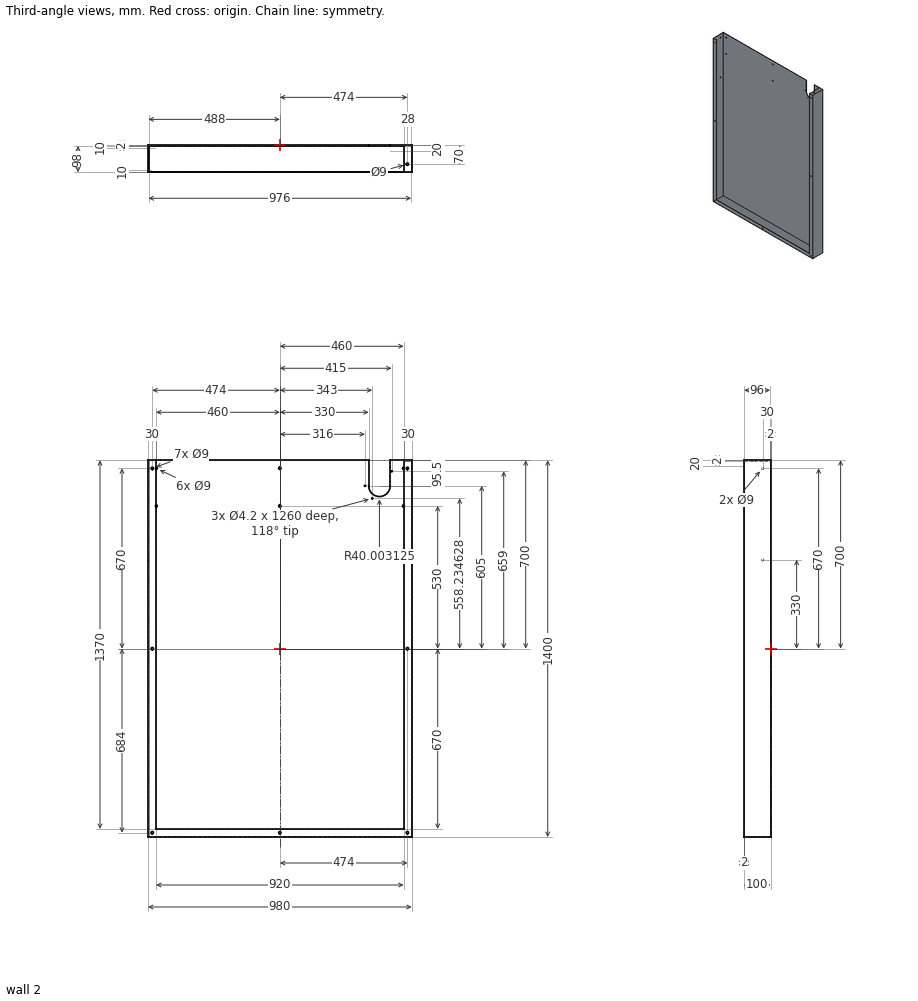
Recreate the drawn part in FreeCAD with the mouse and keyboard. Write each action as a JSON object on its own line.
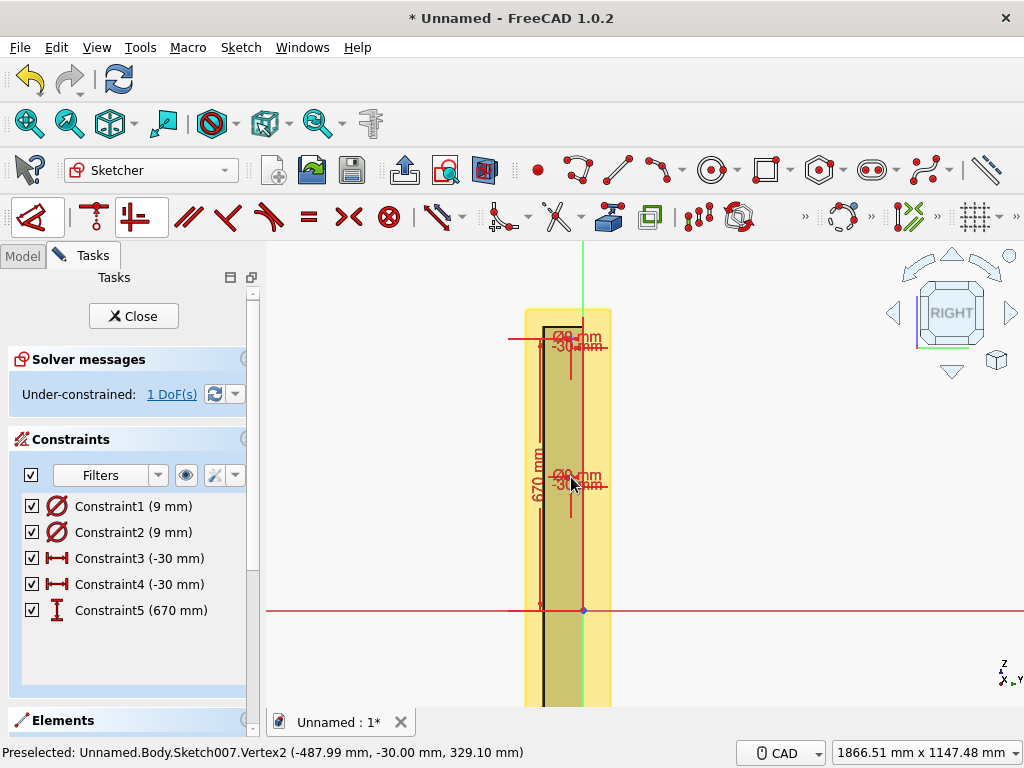
{"action": "key", "text": "i"}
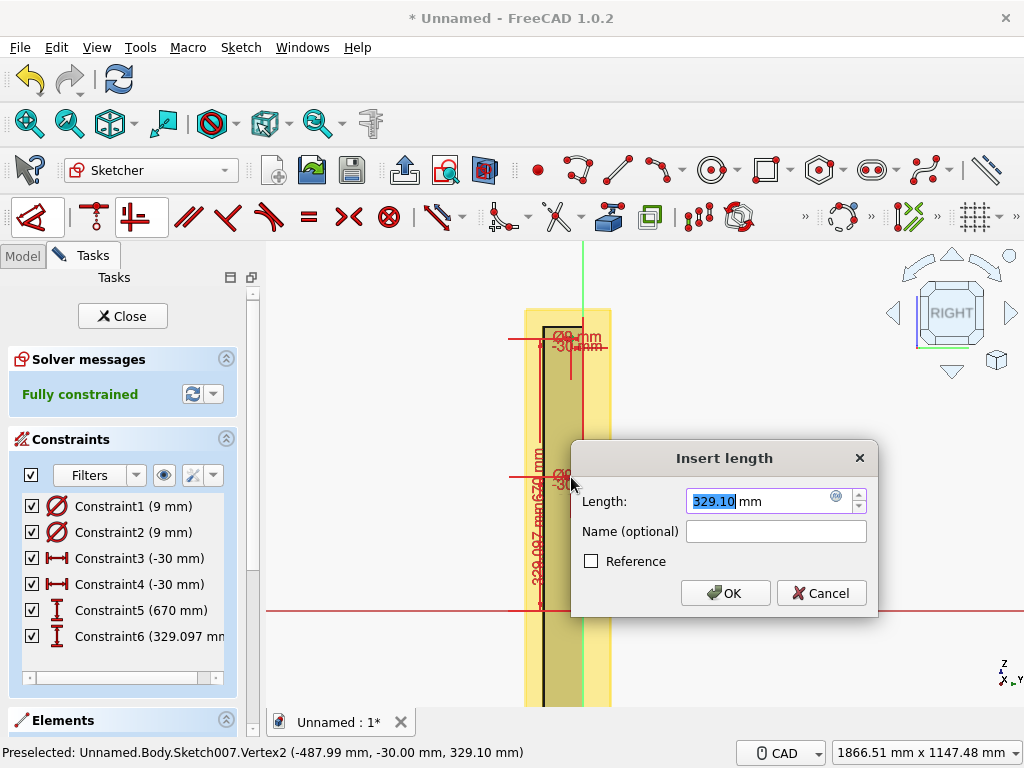
{"action": "type", "text": "330"}
{"action": "key", "text": "Return"}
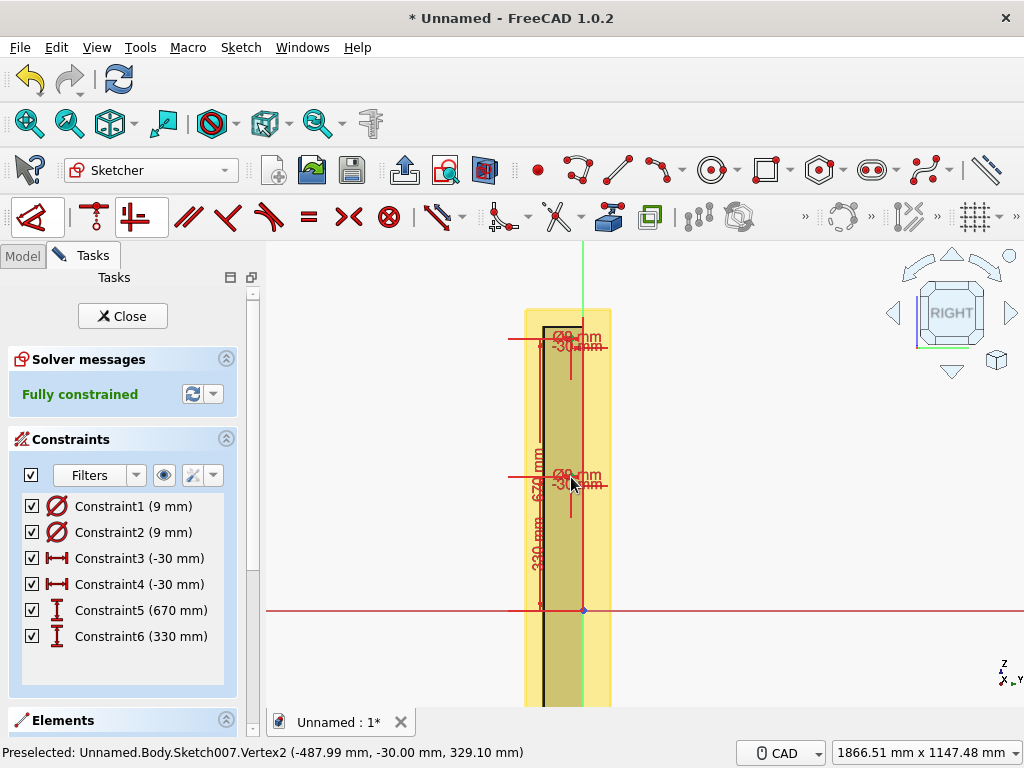
{"action": "left_click", "coordinate": [123, 316]}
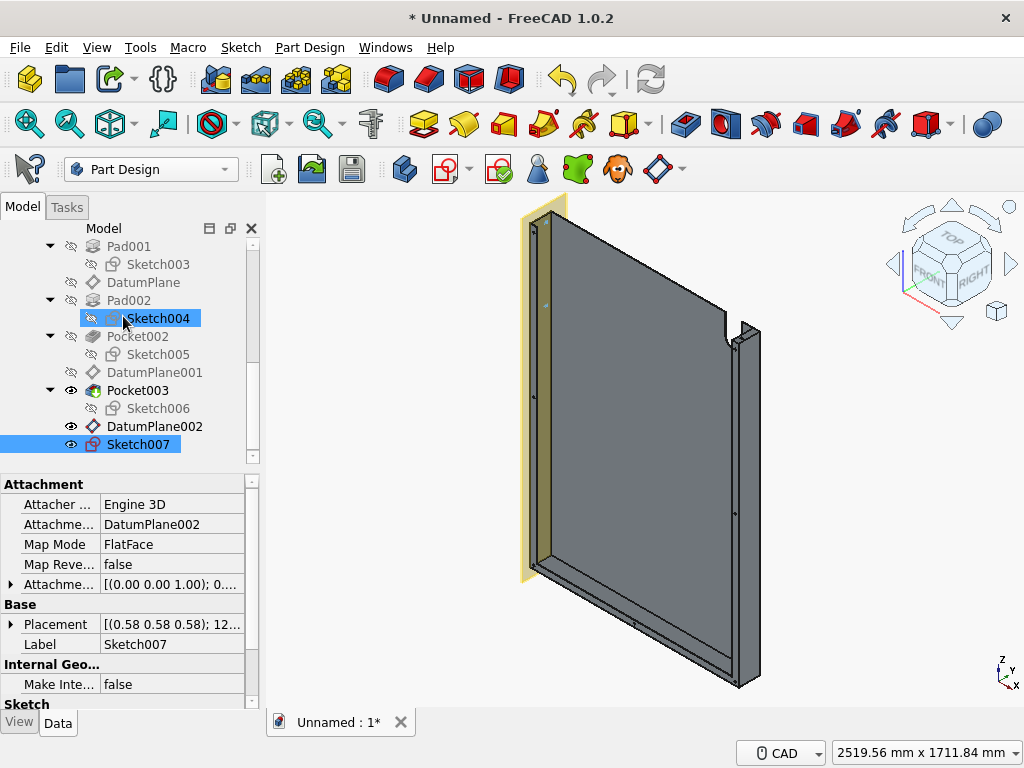
{"action": "left_click", "coordinate": [686, 124]}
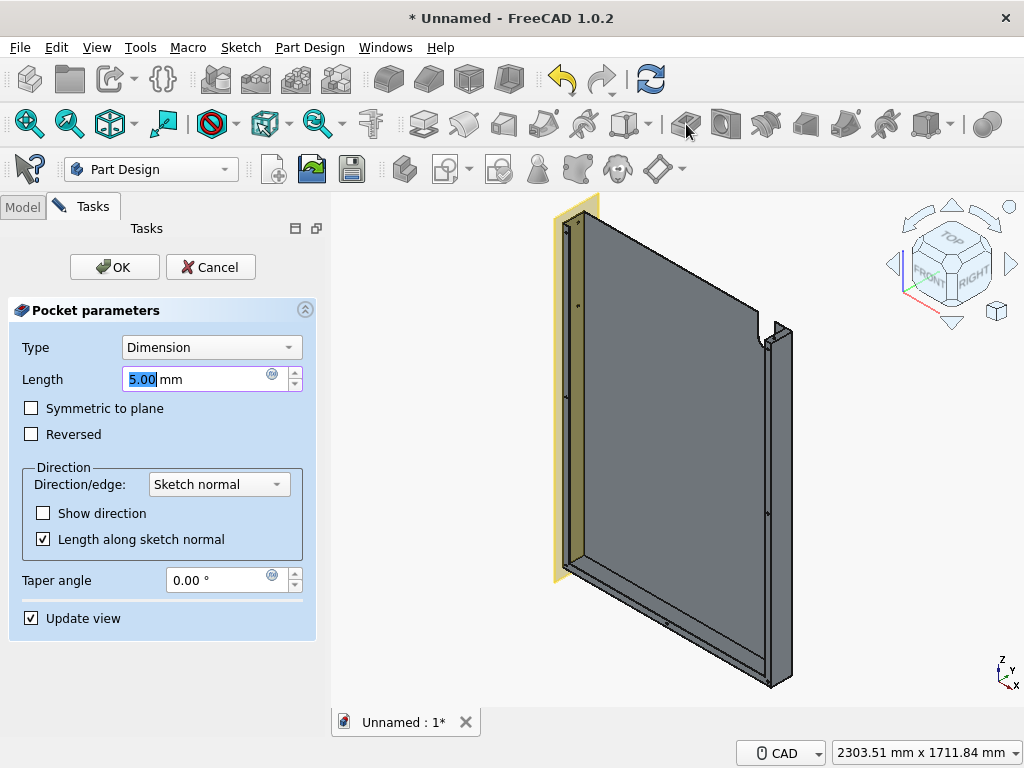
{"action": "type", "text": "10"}
{"action": "key", "text": "Tab"}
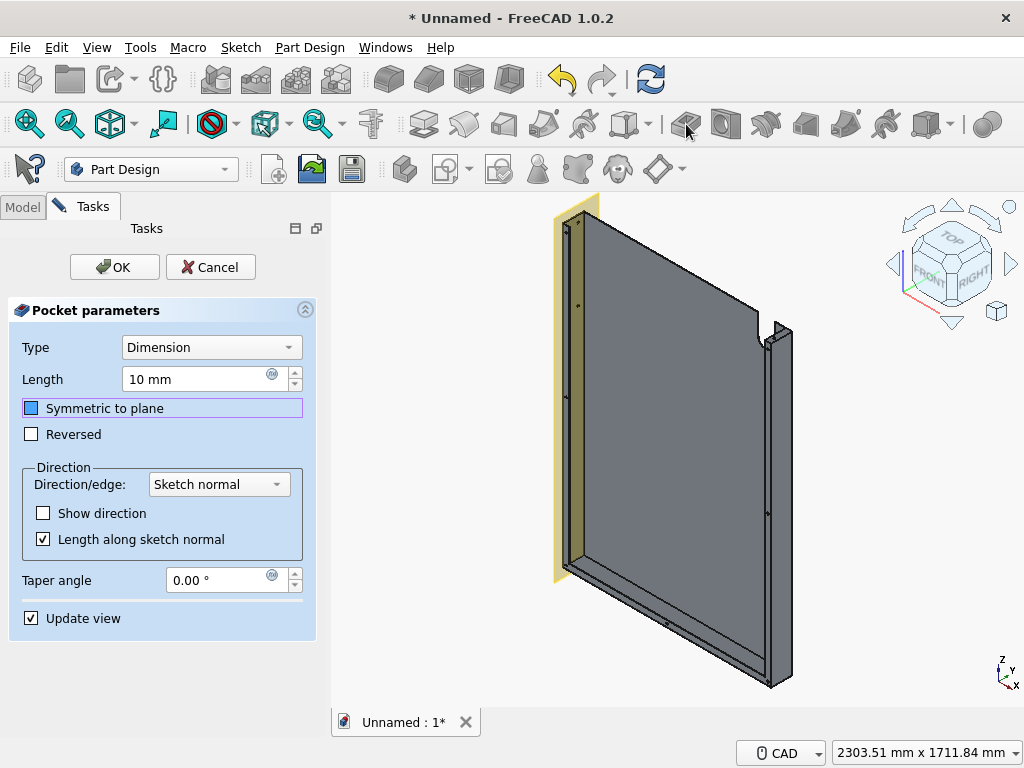
{"action": "left_click", "coordinate": [115, 267]}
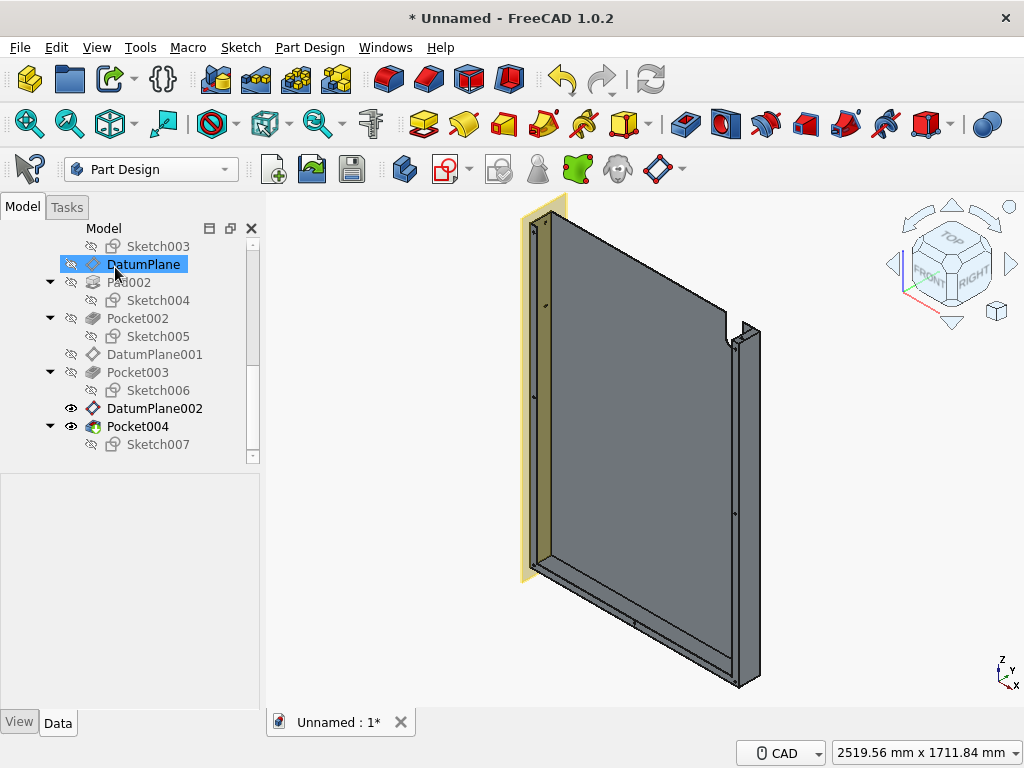
{"action": "left_click", "coordinate": [116, 408]}
{"action": "key", "text": "space"}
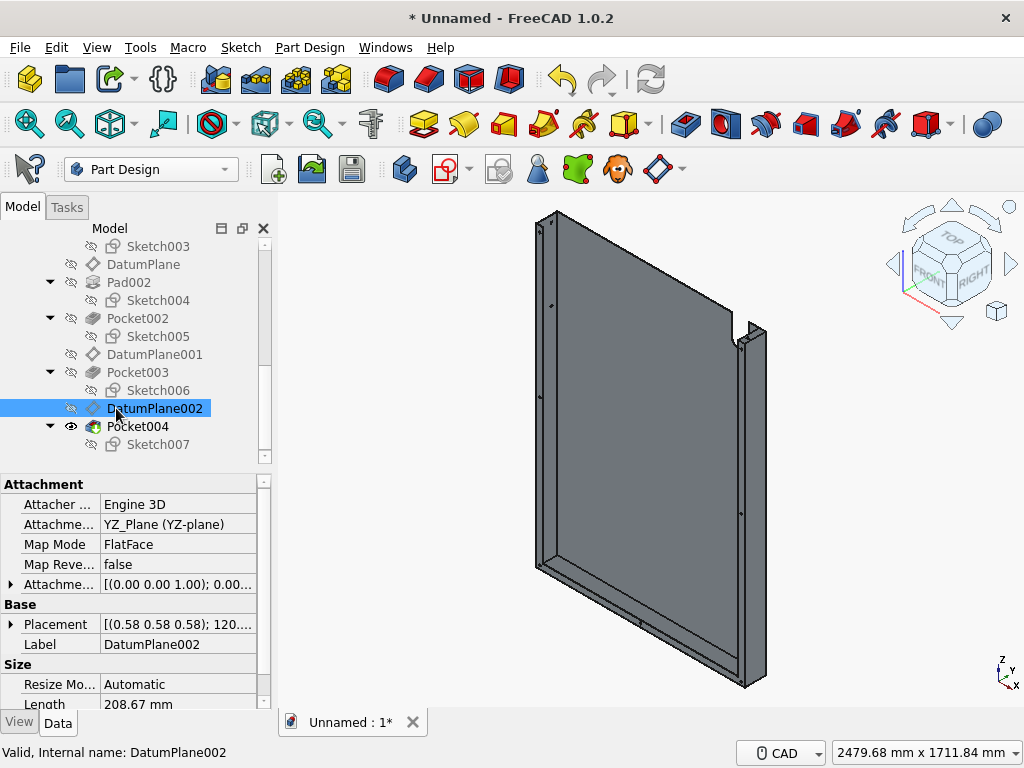
{"action": "key", "text": "4"}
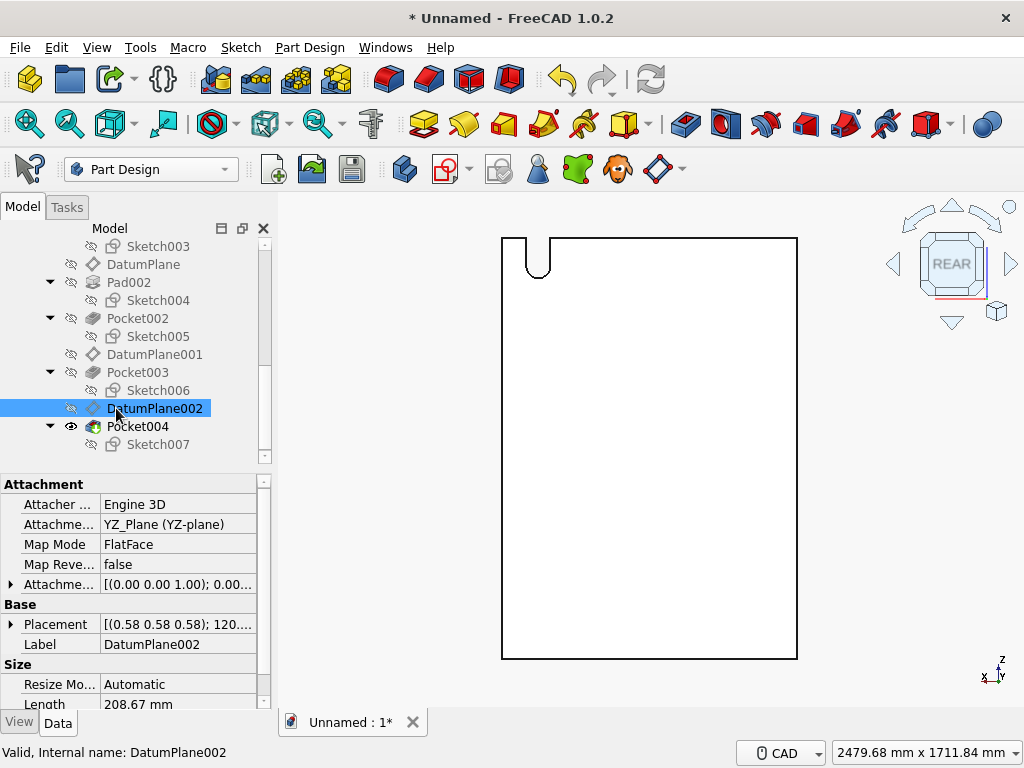
{"action": "left_click", "coordinate": [650, 387]}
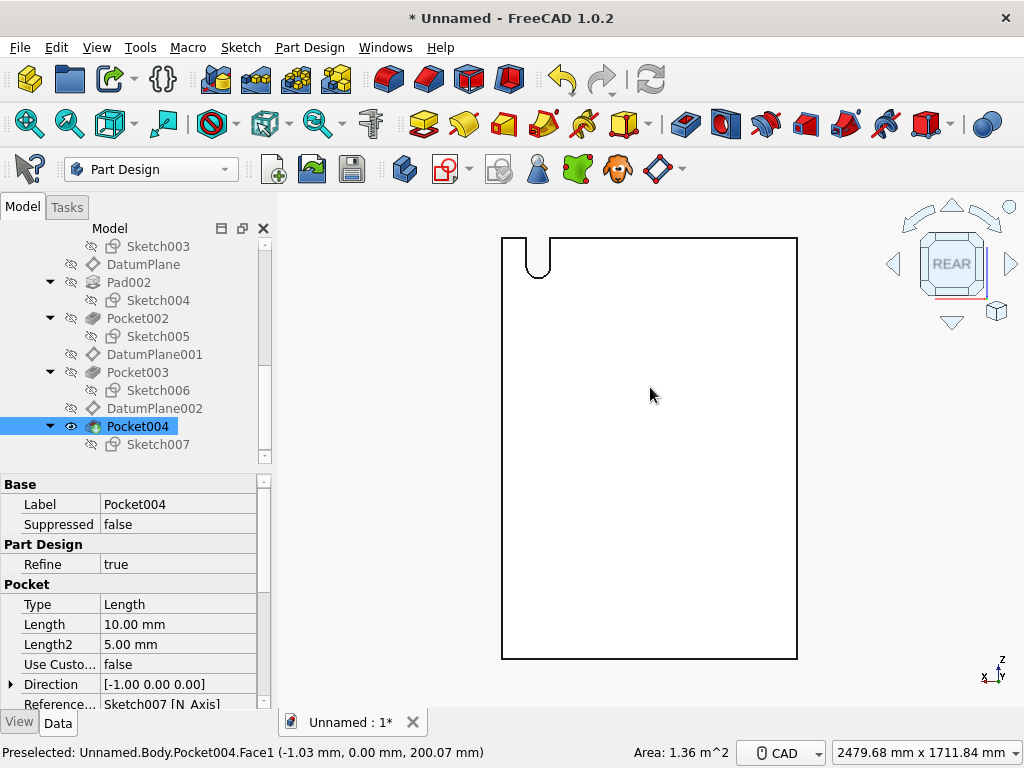
{"action": "left_click", "coordinate": [446, 170]}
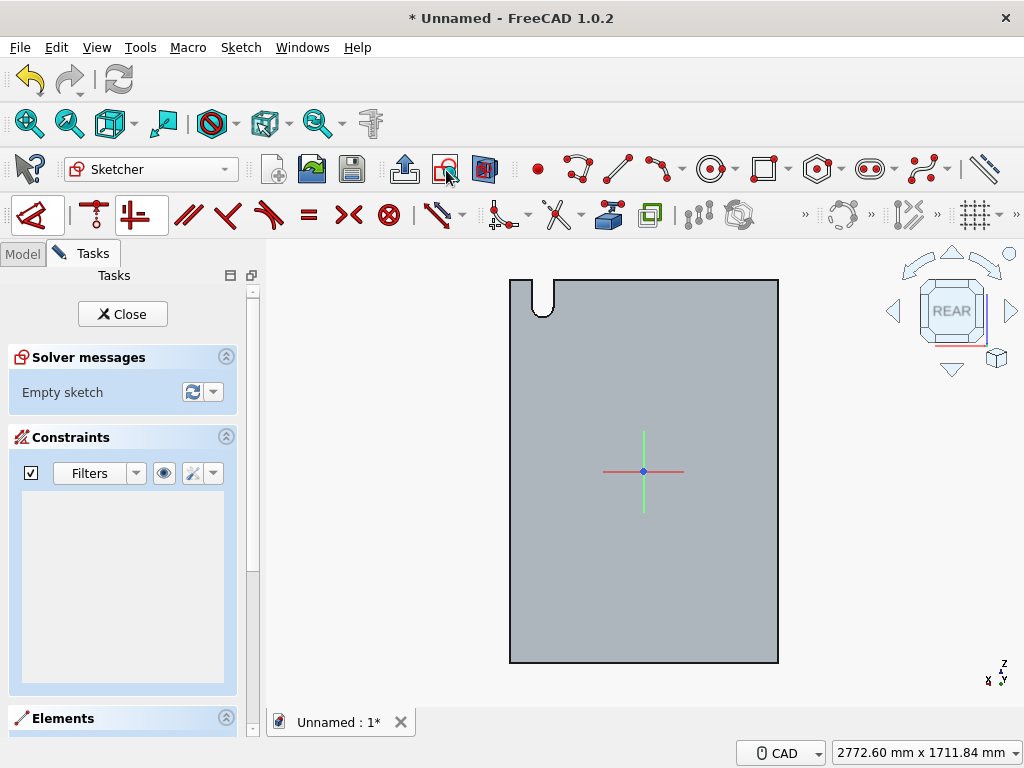
{"action": "scroll", "coordinate": [781, 267], "scroll_direction": "up", "scroll_amount": 2}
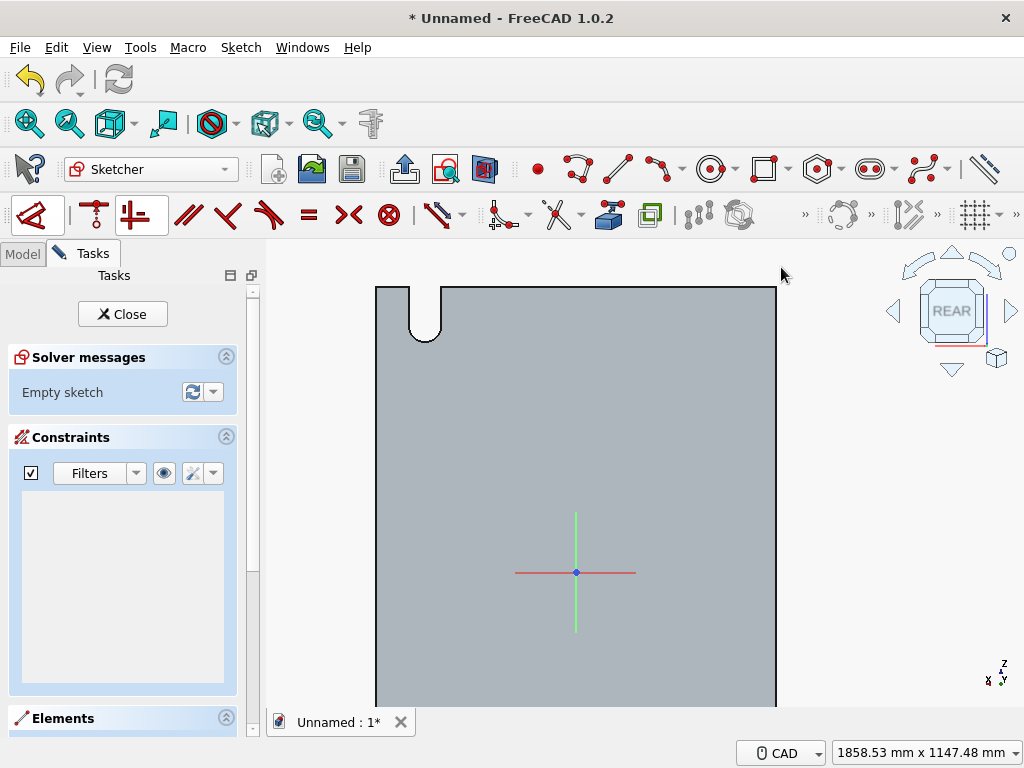
{"action": "left_click", "coordinate": [712, 170]}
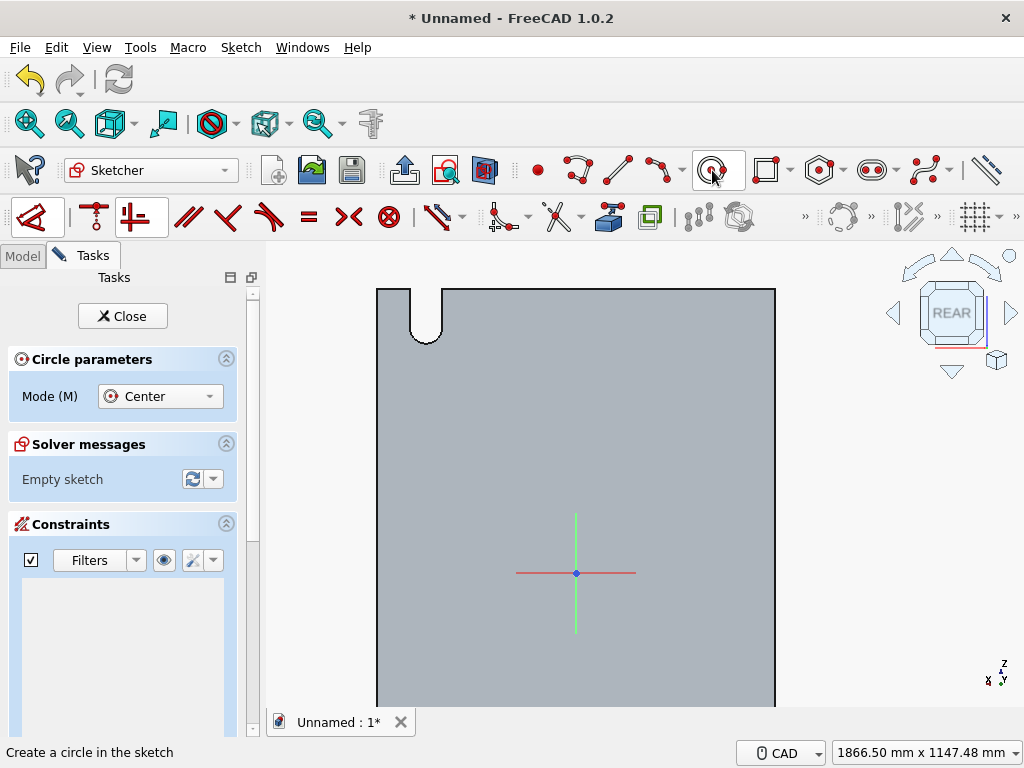
{"action": "scroll", "coordinate": [763, 301], "scroll_direction": "up", "scroll_amount": 13}